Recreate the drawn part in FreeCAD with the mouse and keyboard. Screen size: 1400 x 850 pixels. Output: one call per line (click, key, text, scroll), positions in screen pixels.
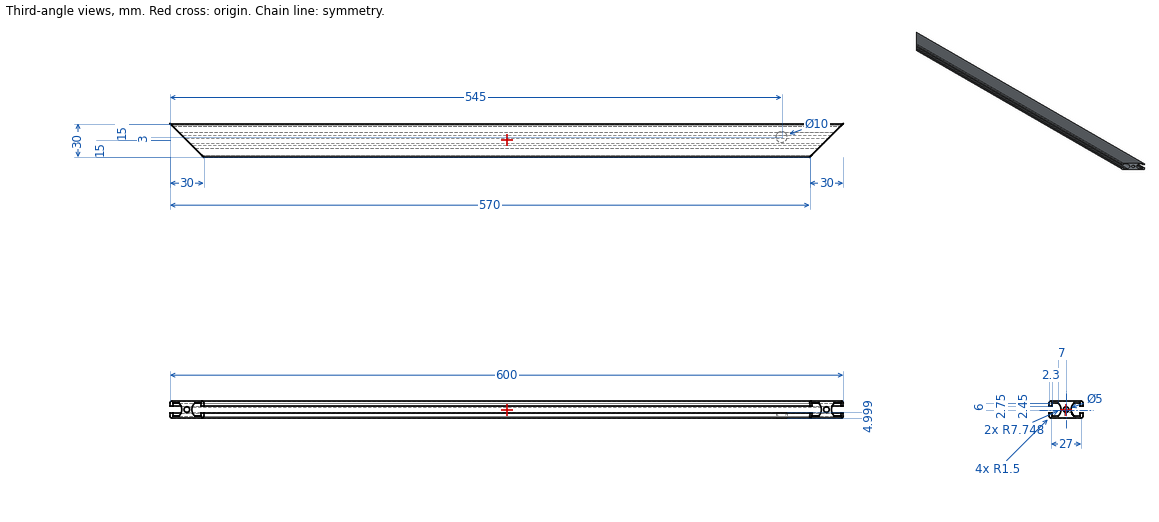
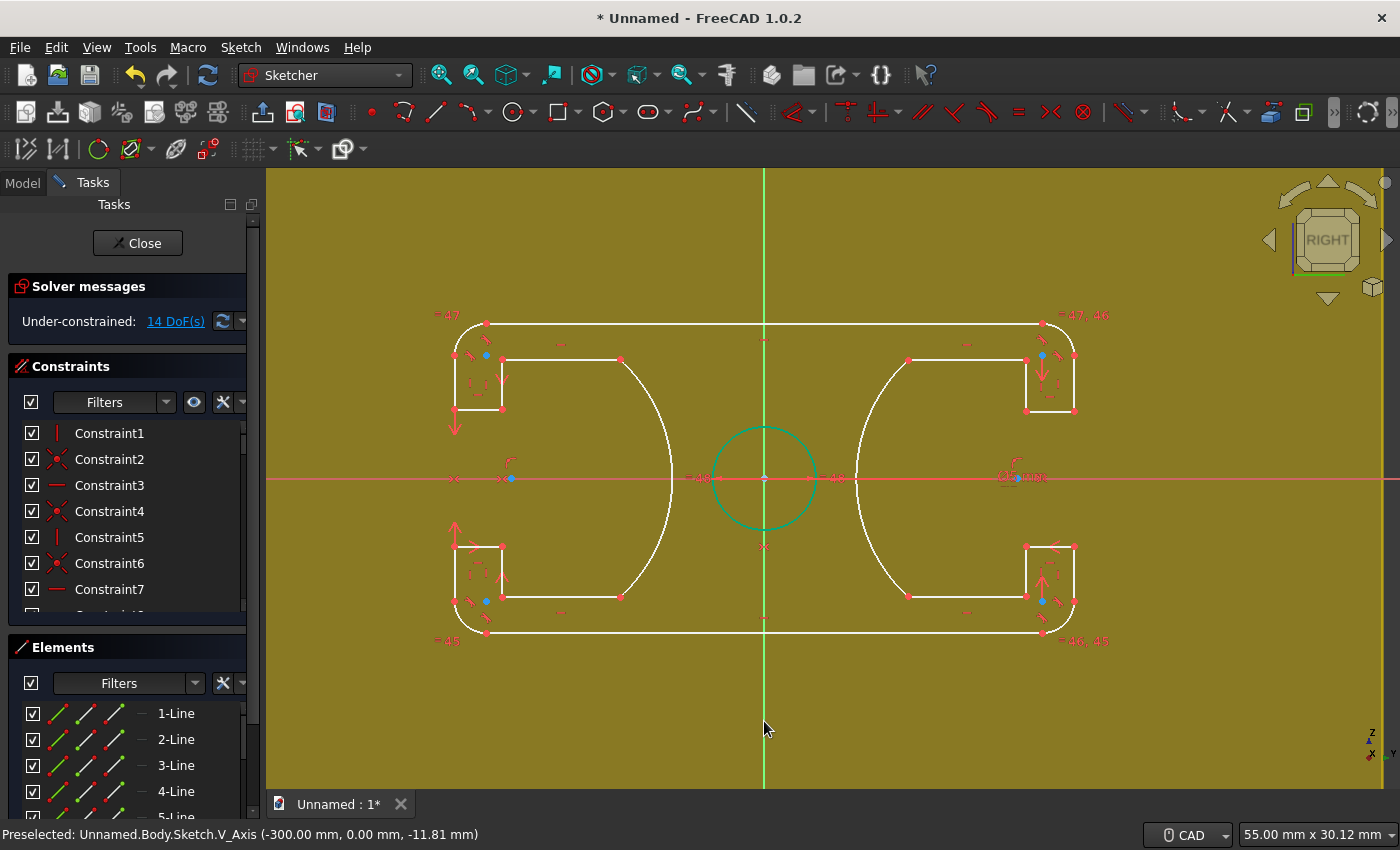
click(502, 597)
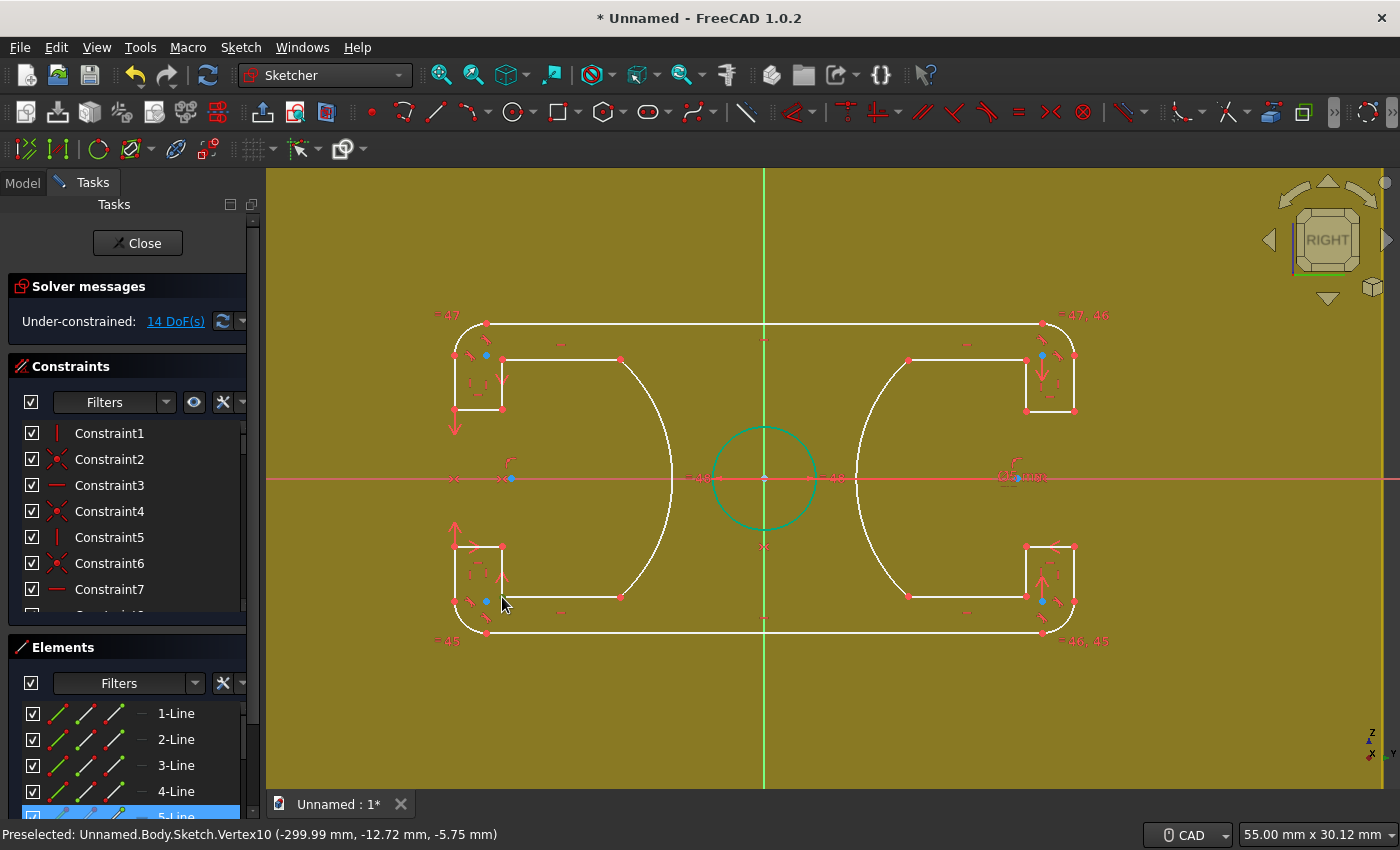
click(1026, 597)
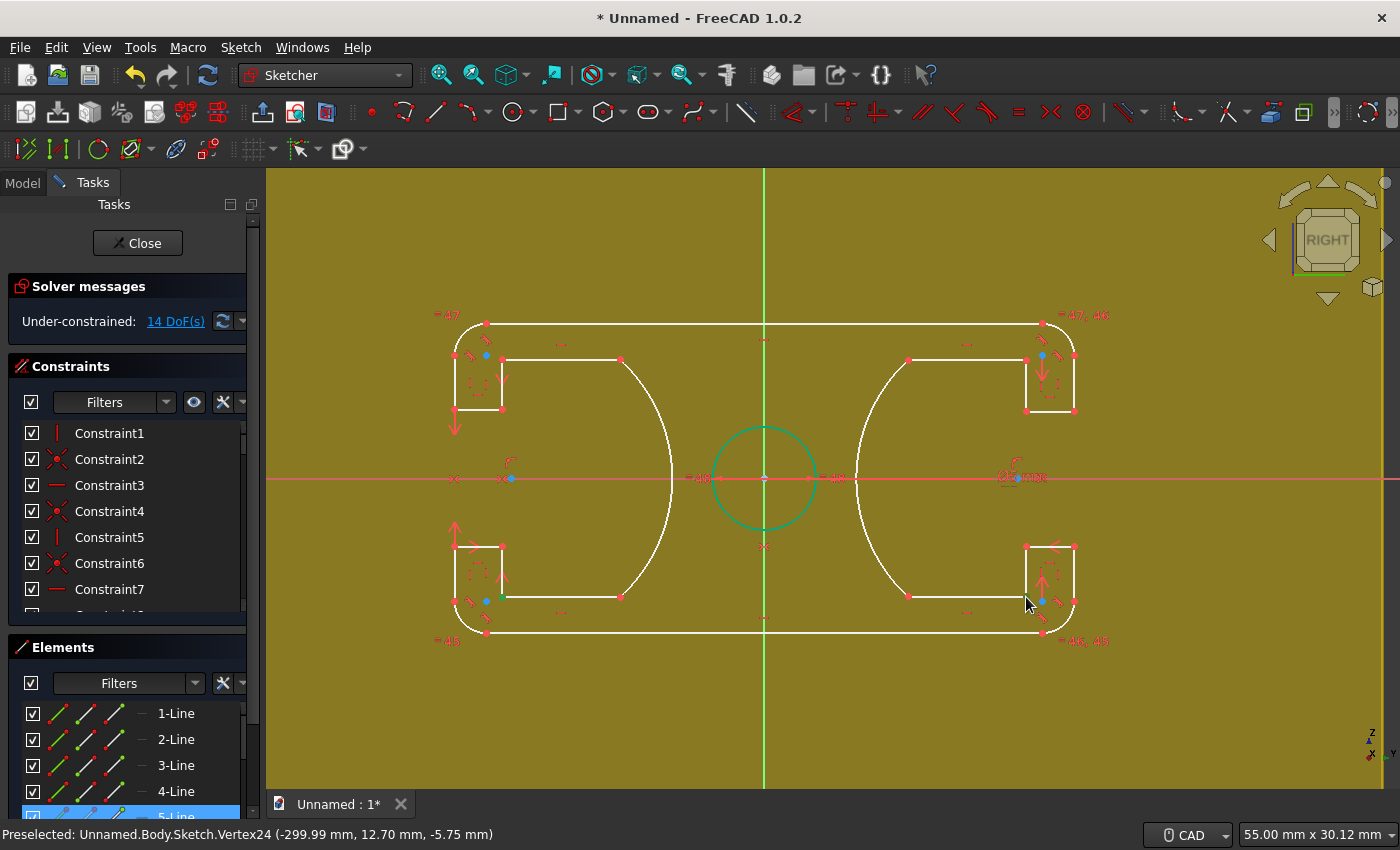
click(764, 721)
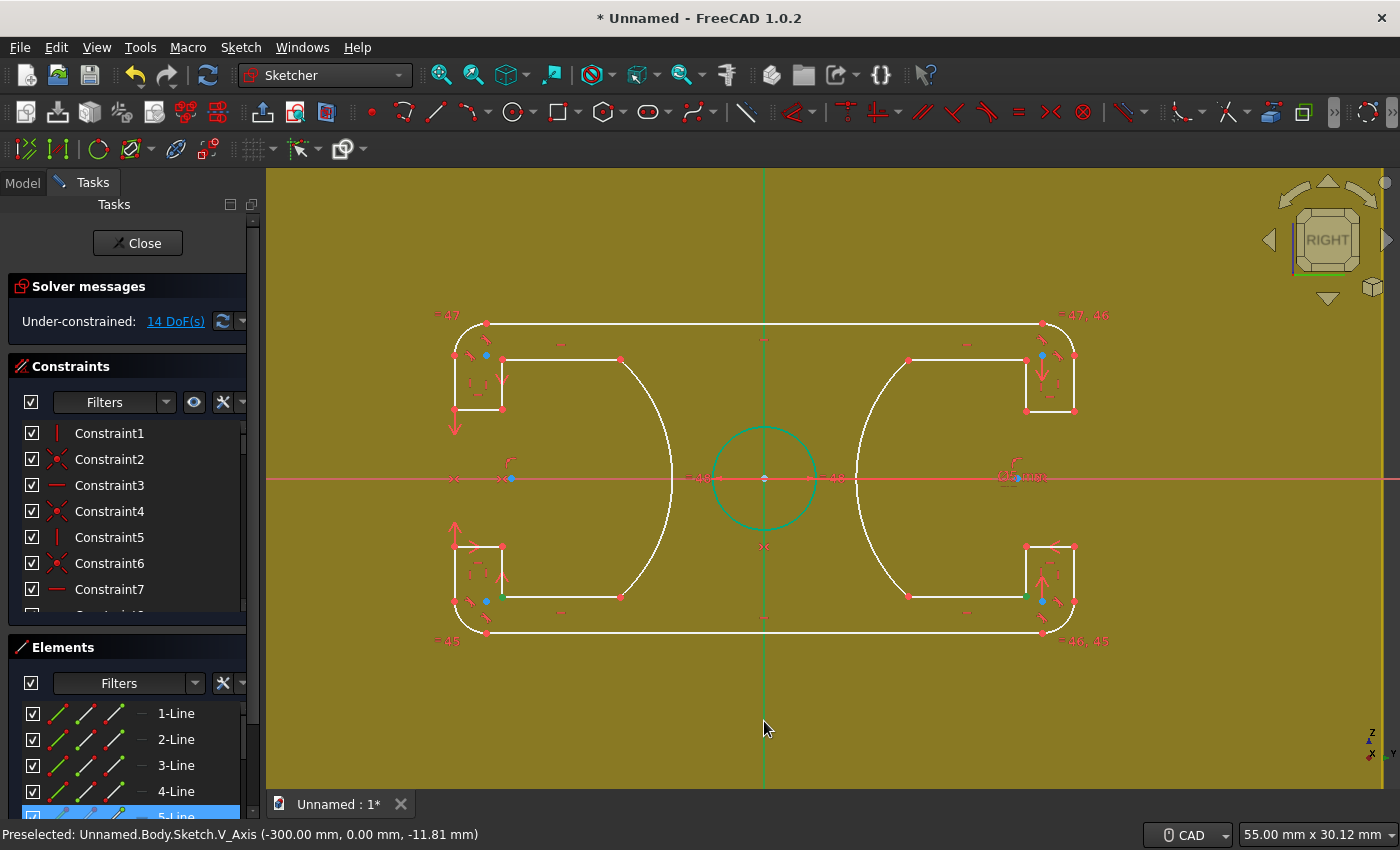
key(s)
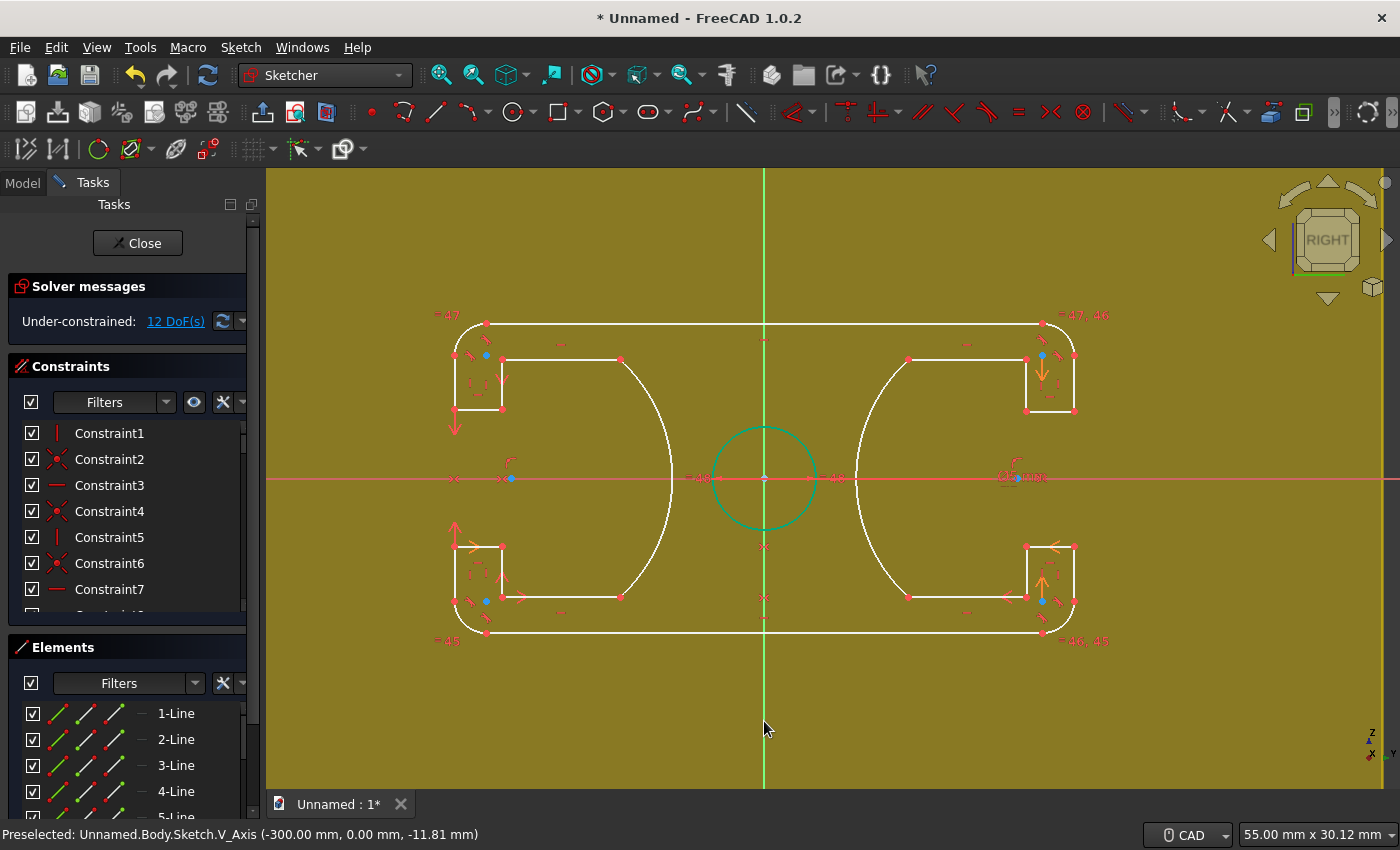
click(620, 360)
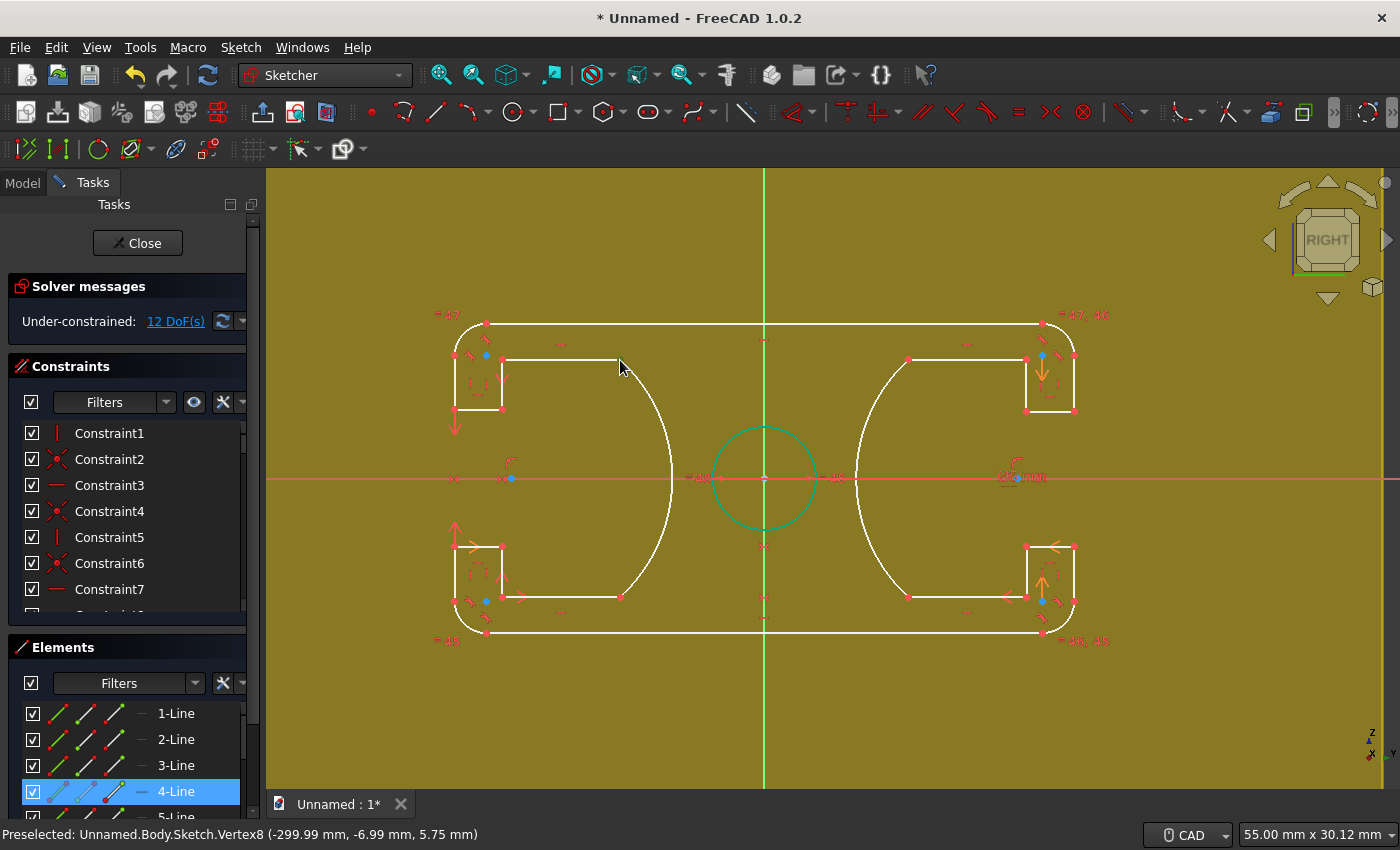
click(908, 360)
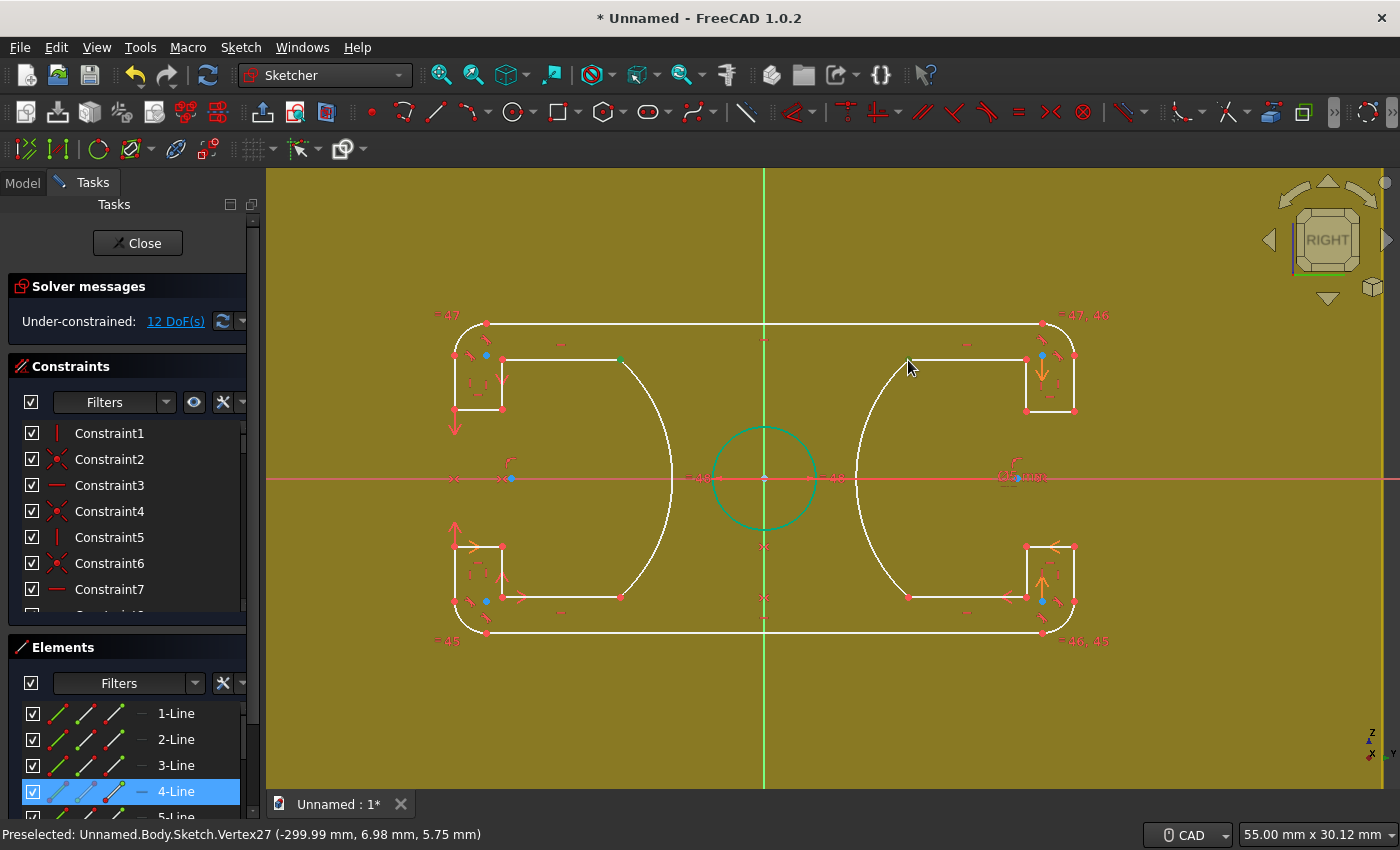
click(764, 721)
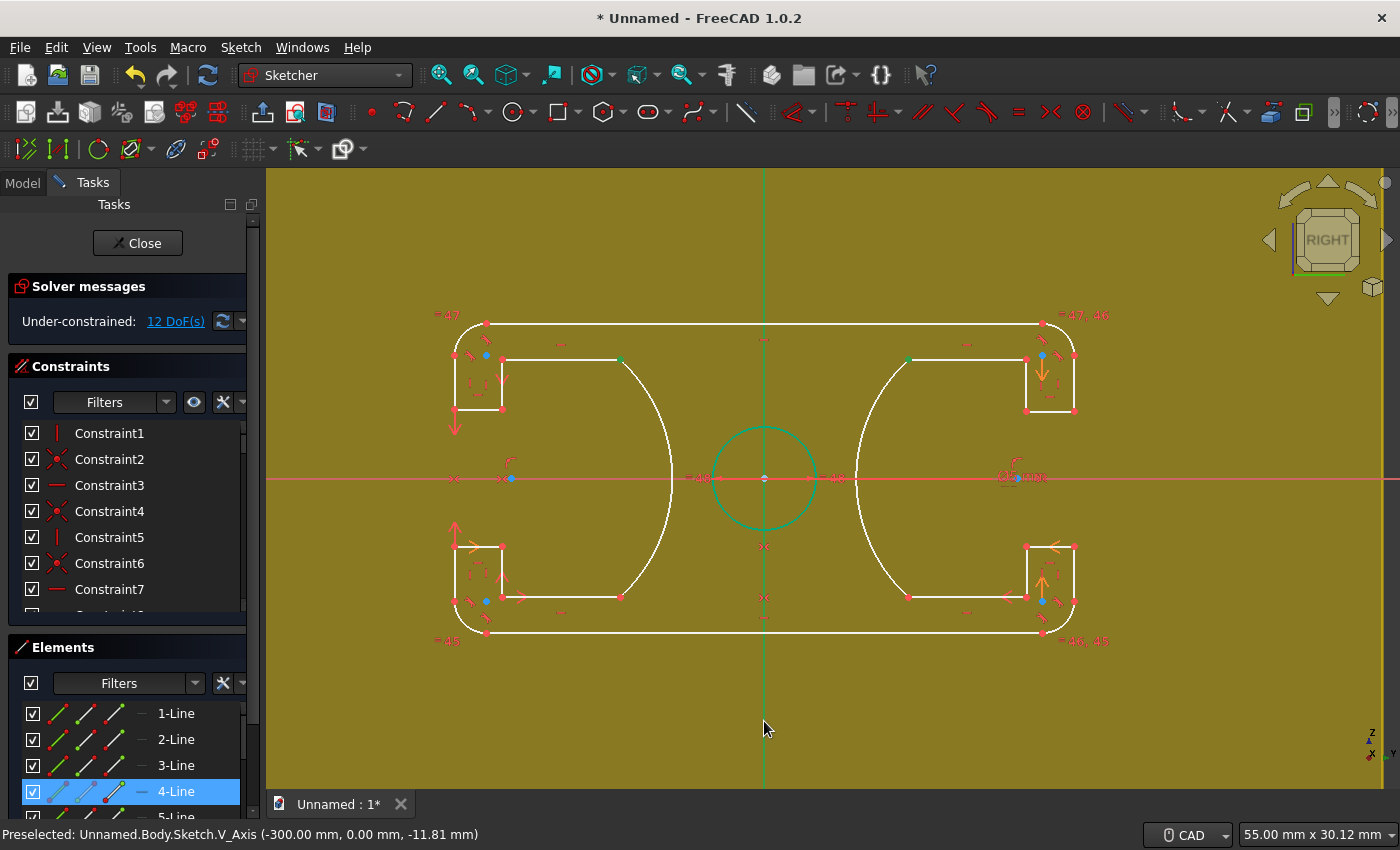
key(s)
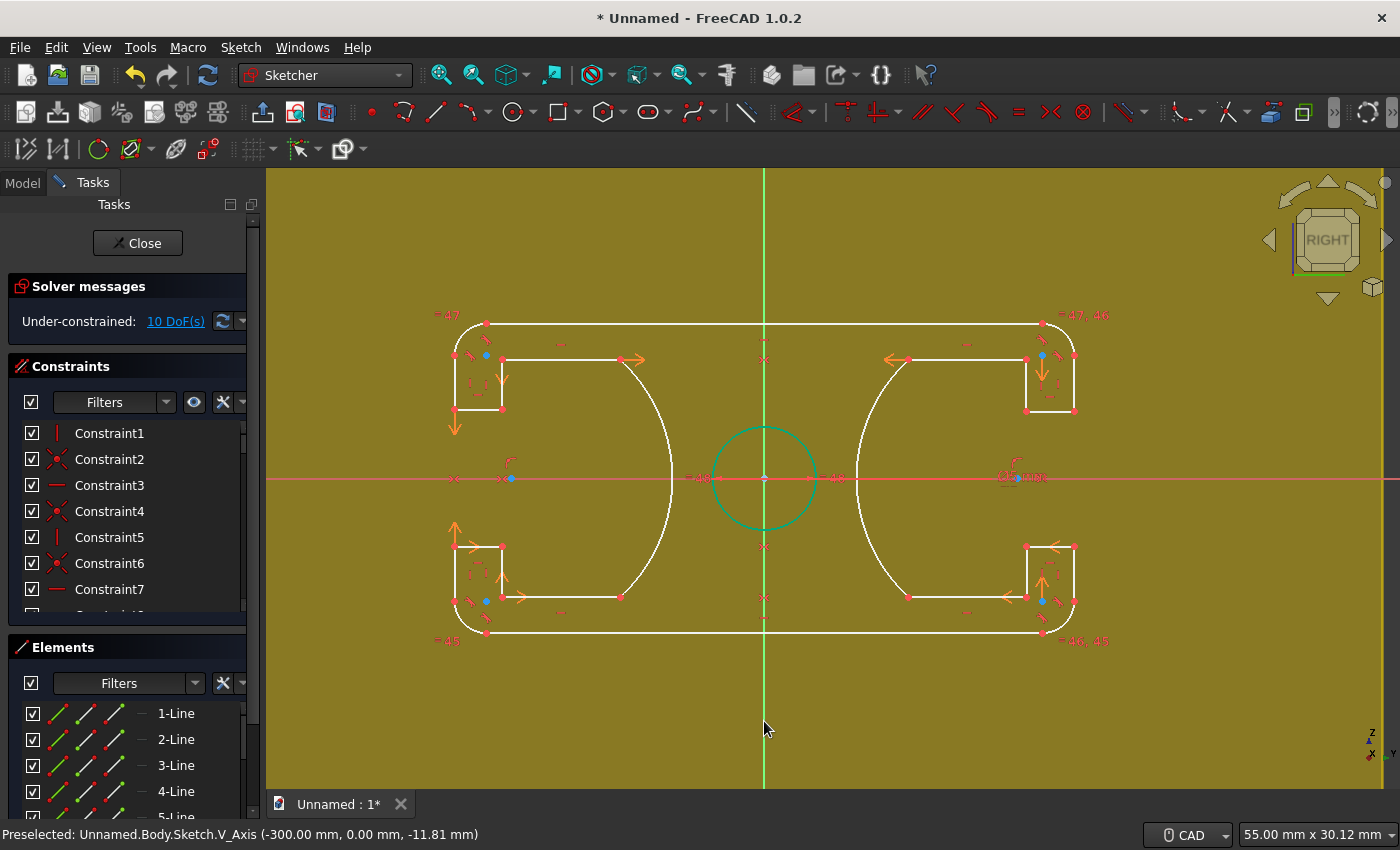
click(502, 410)